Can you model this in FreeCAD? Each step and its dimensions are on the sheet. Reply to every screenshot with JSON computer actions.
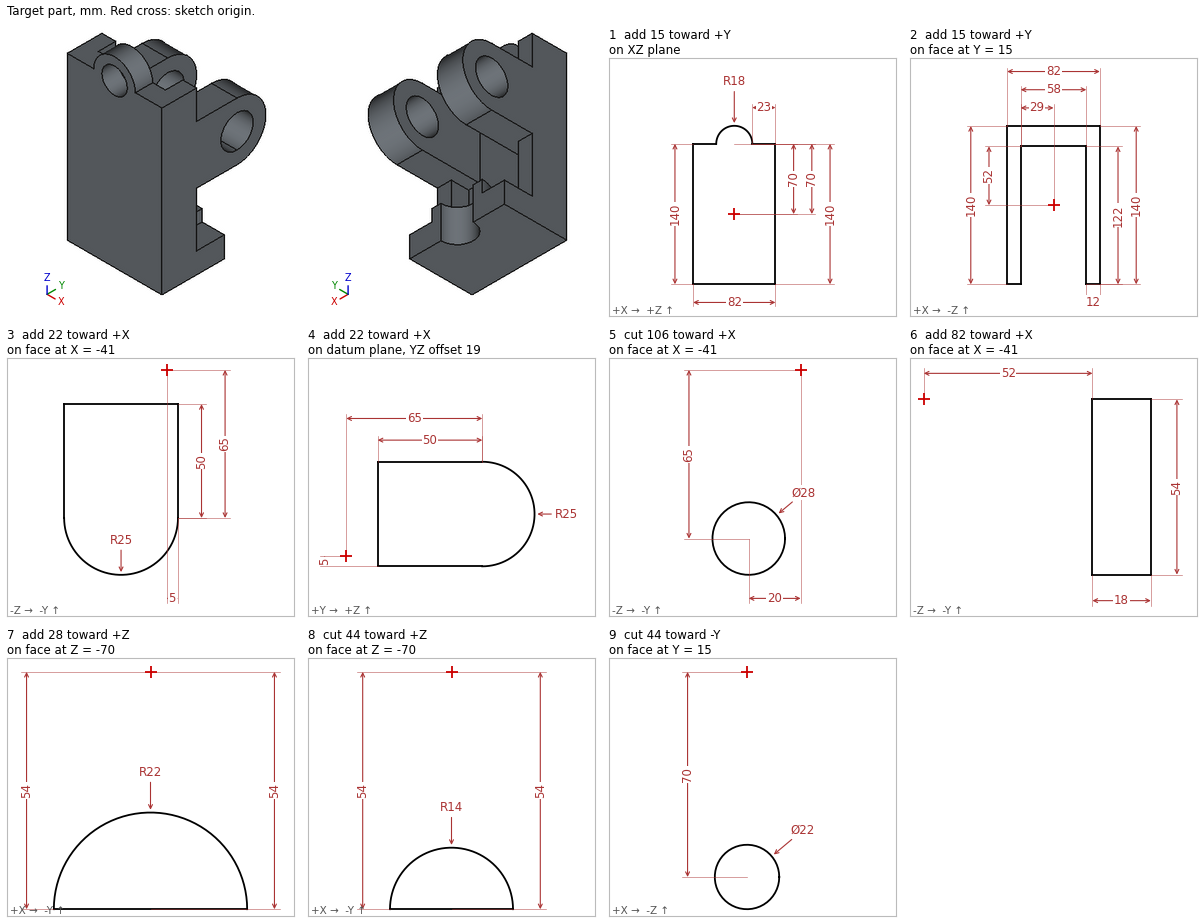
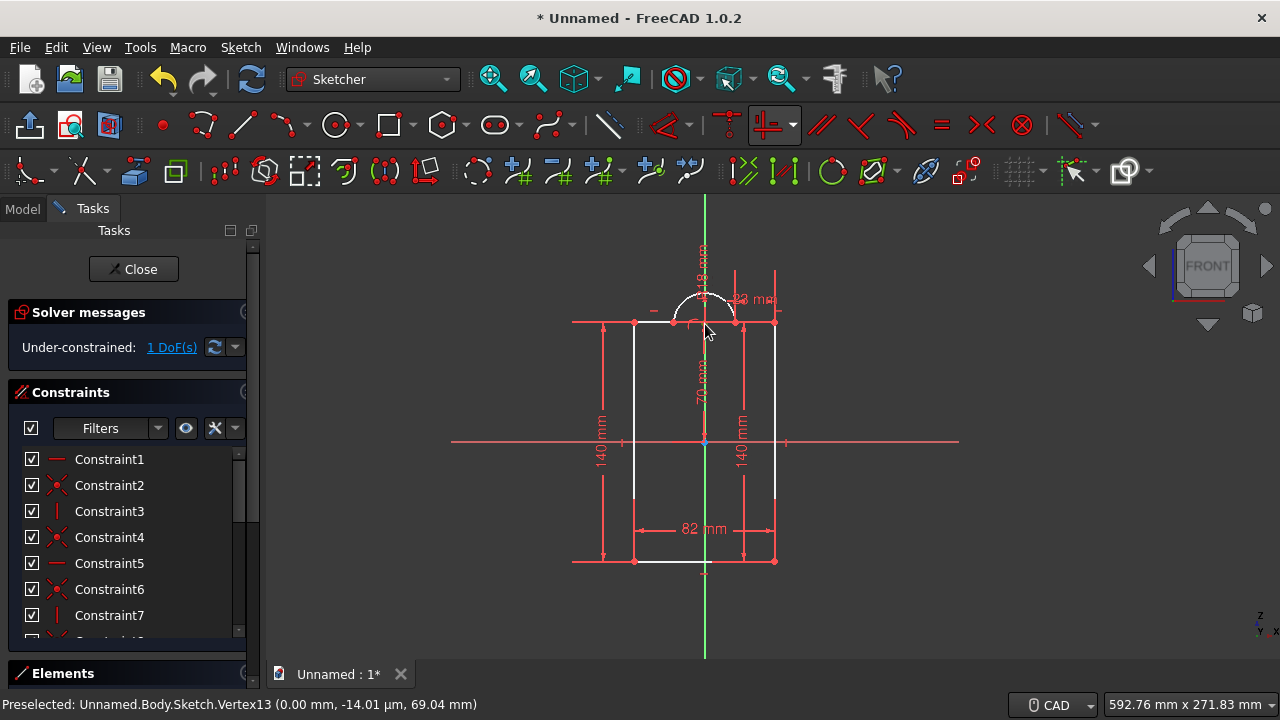
{"action": "left_click", "coordinate": [692, 126]}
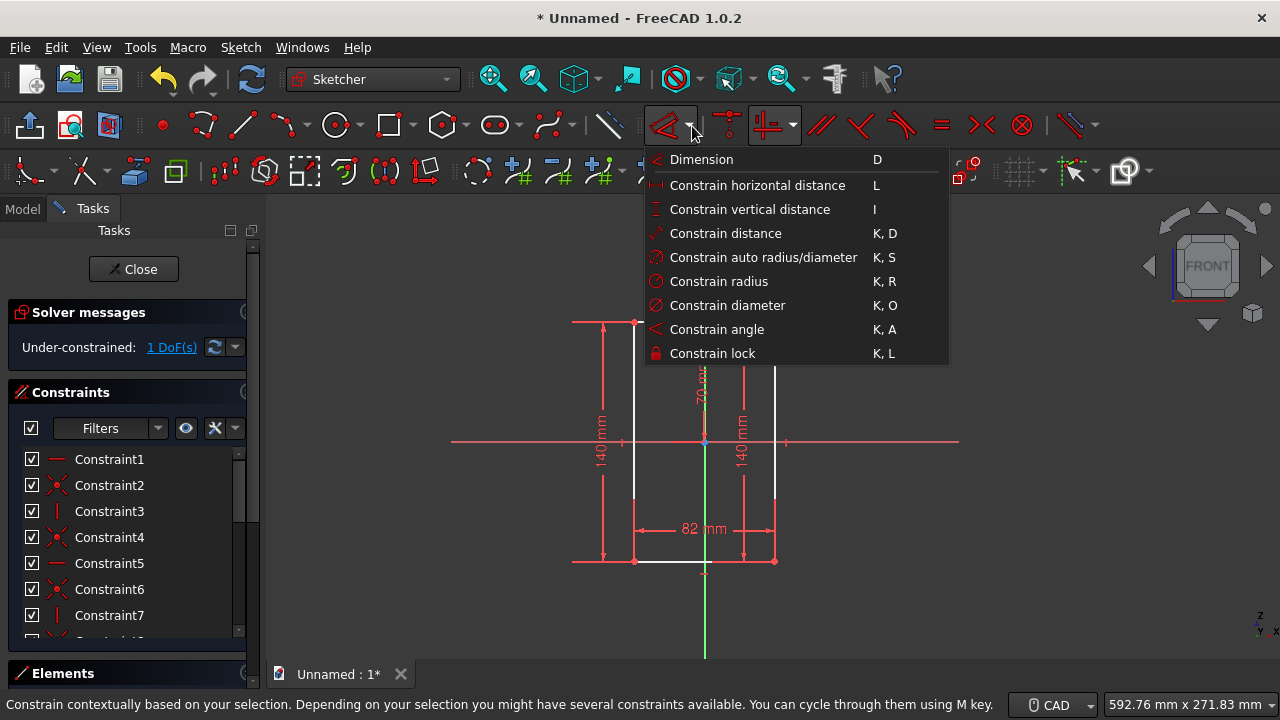
{"action": "left_click", "coordinate": [797, 209]}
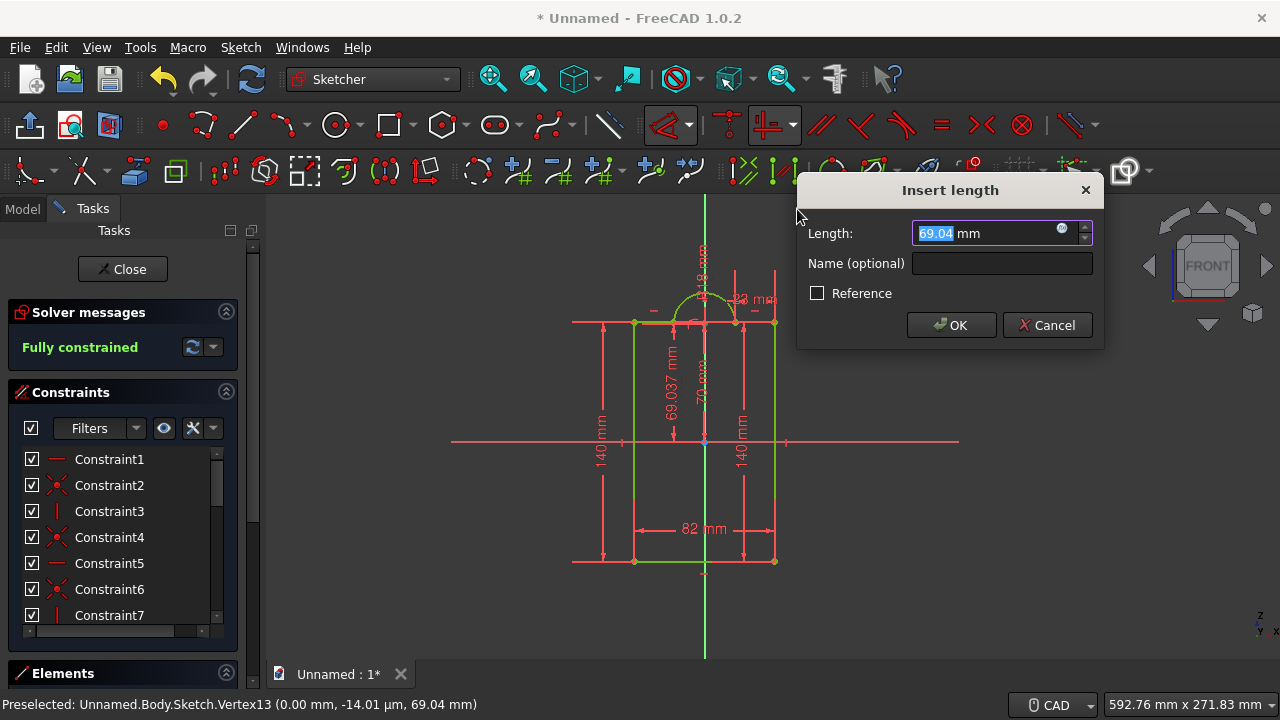
{"action": "type", "text": "70"}
{"action": "key", "text": "Return"}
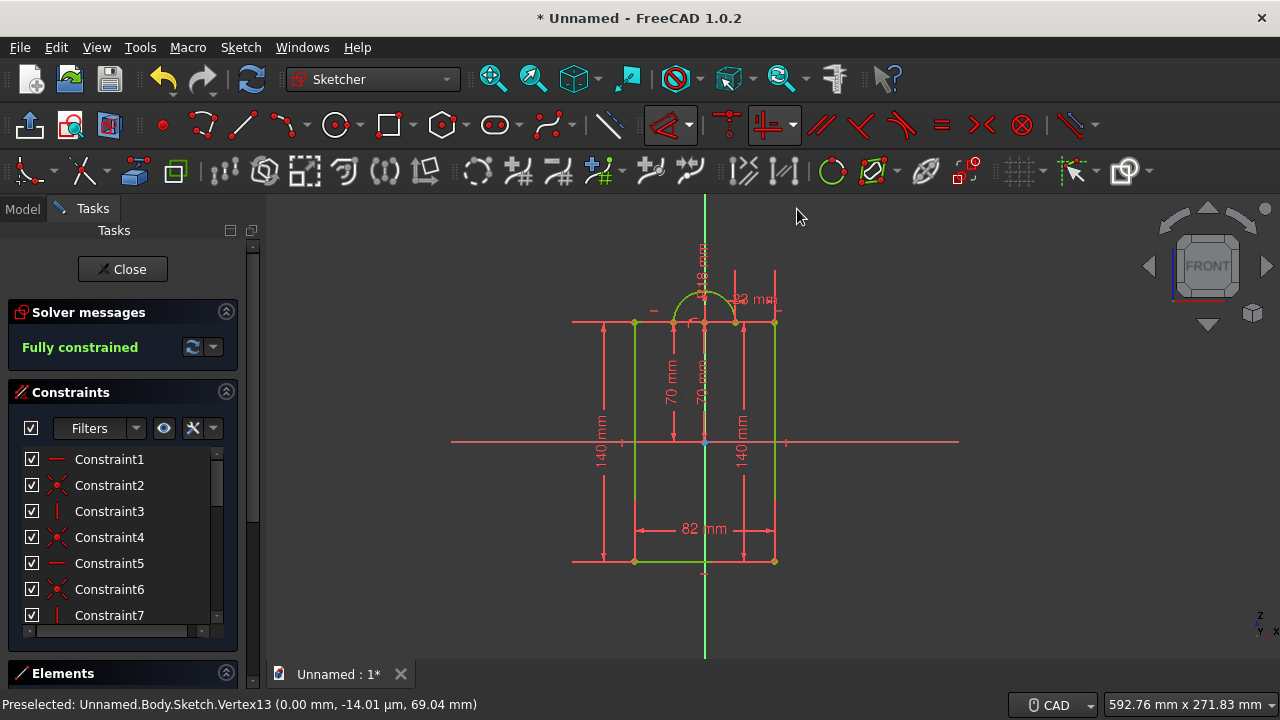
{"action": "left_click", "coordinate": [123, 269]}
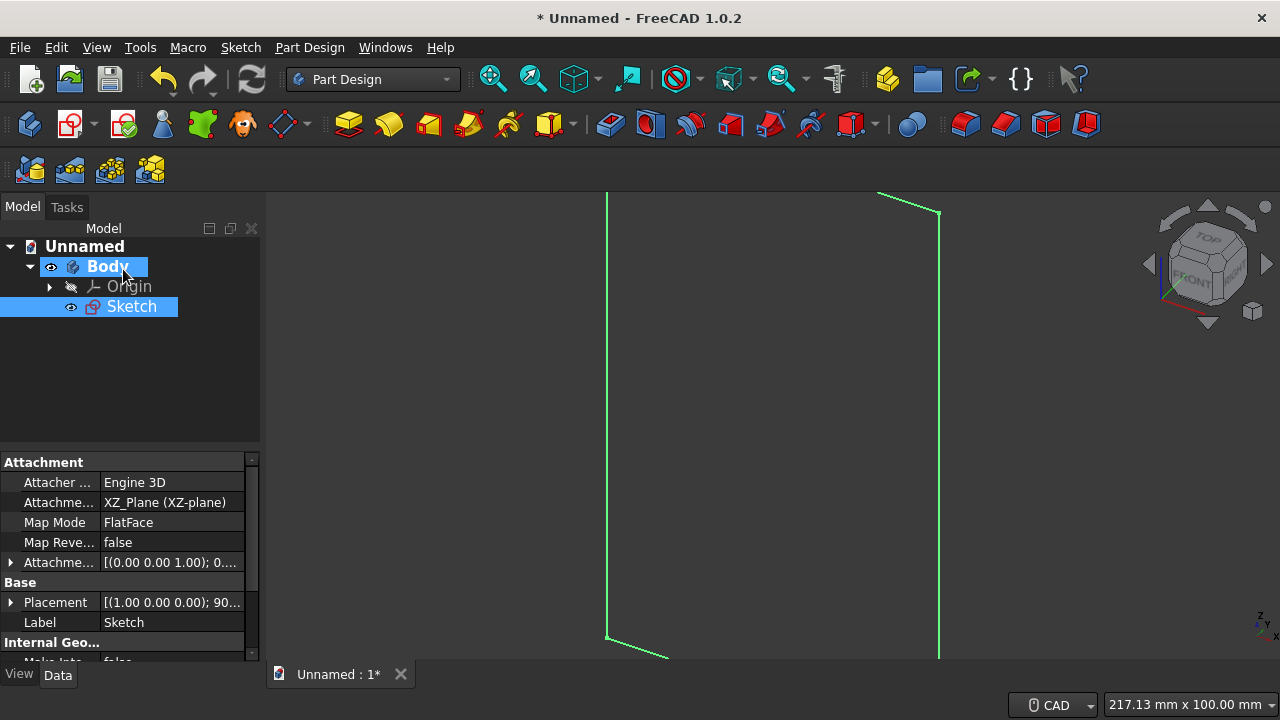
{"action": "left_click", "coordinate": [350, 124]}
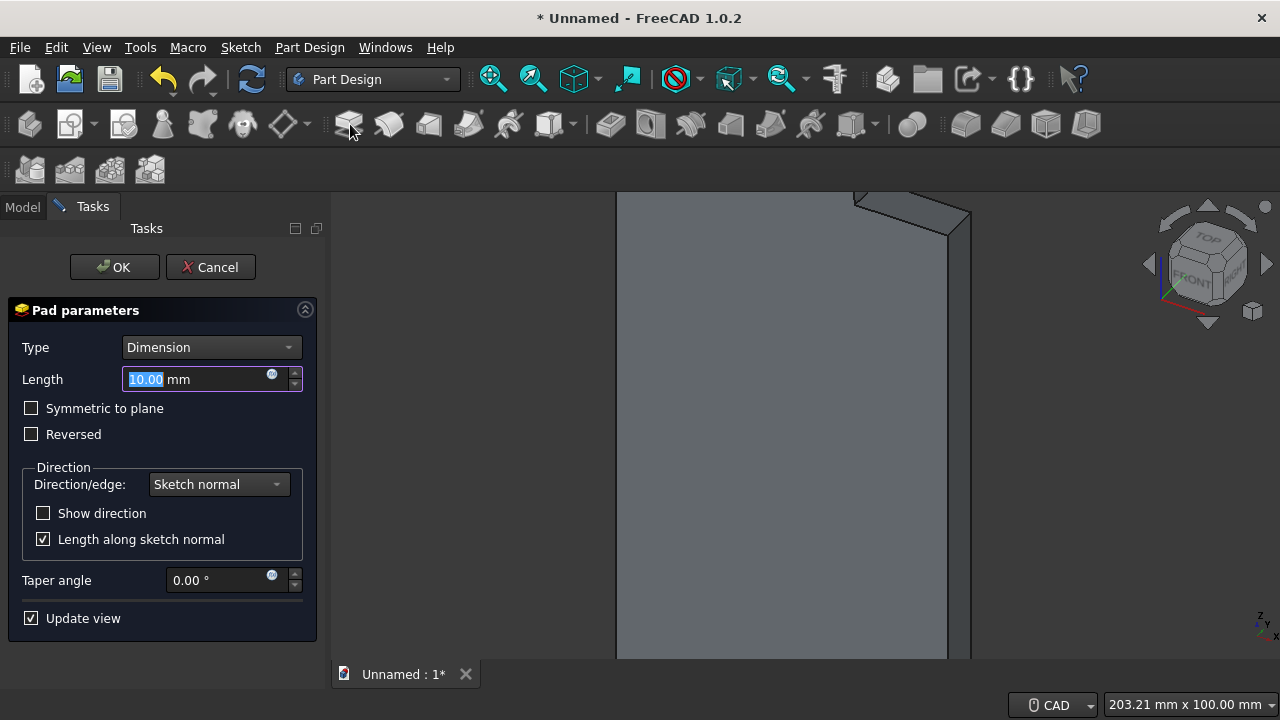
{"action": "type", "text": "15"}
{"action": "key", "text": "Tab"}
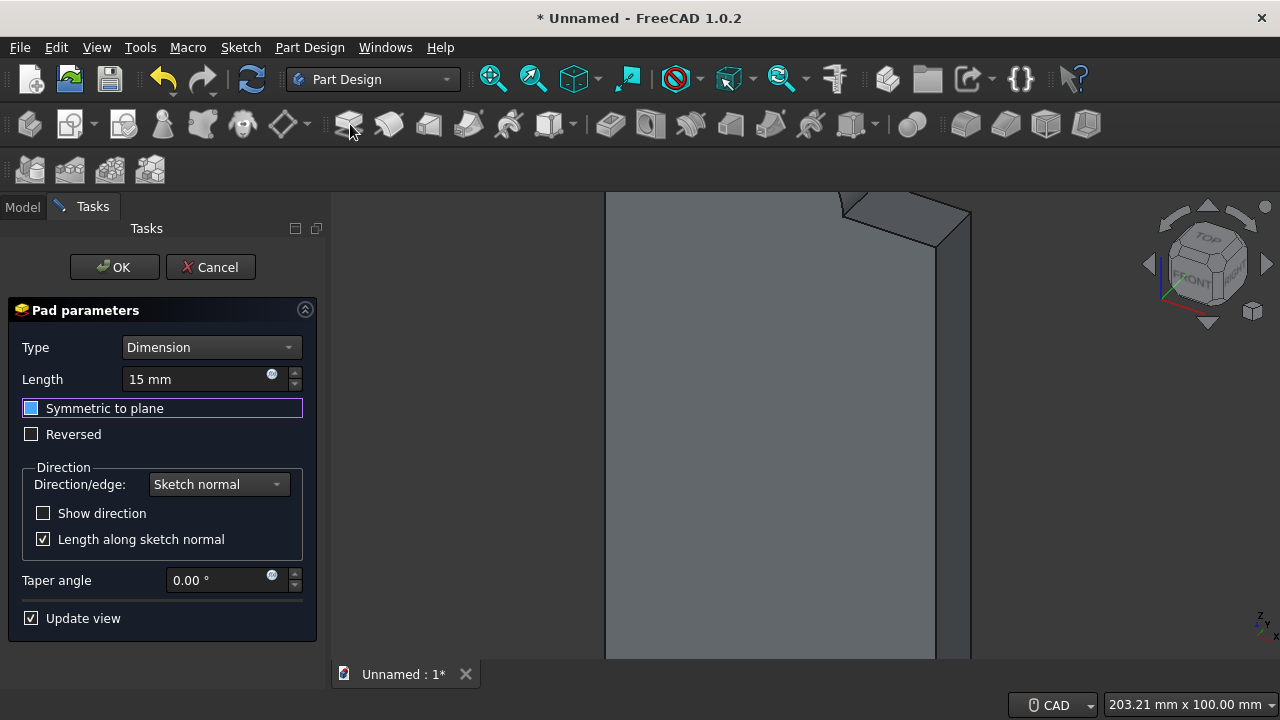
{"action": "left_click", "coordinate": [30, 434]}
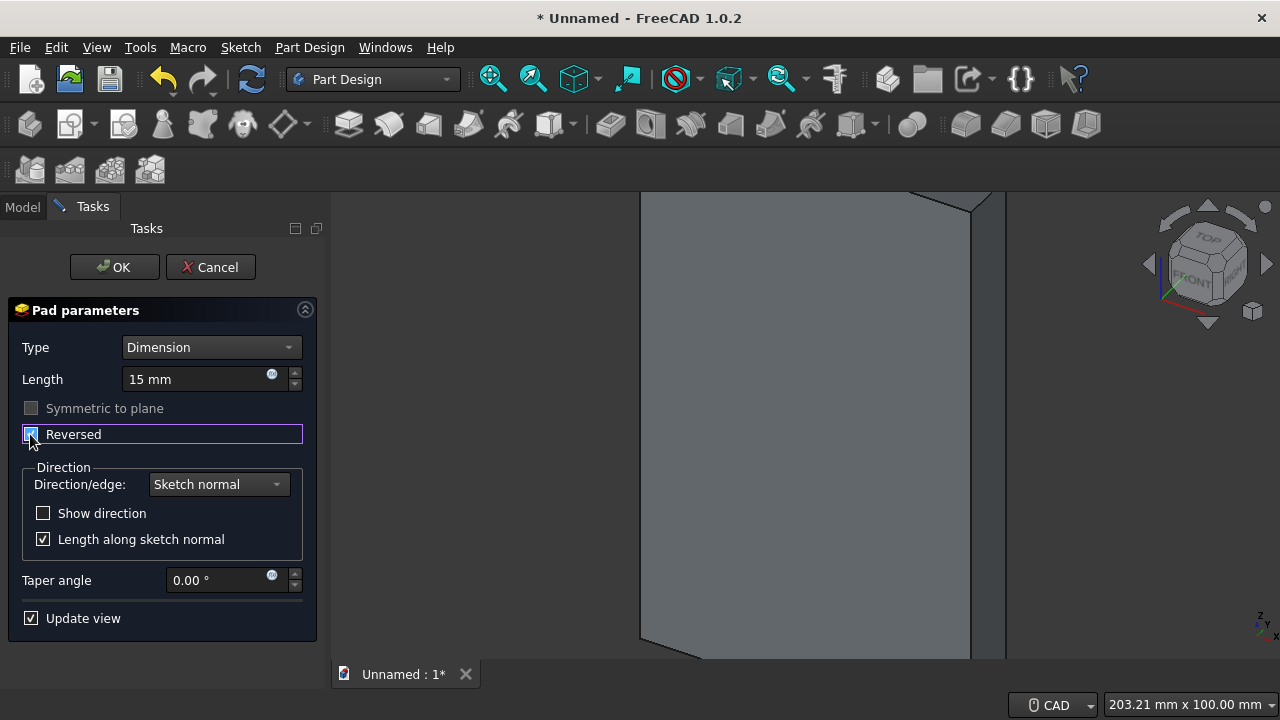
{"action": "left_click", "coordinate": [115, 267]}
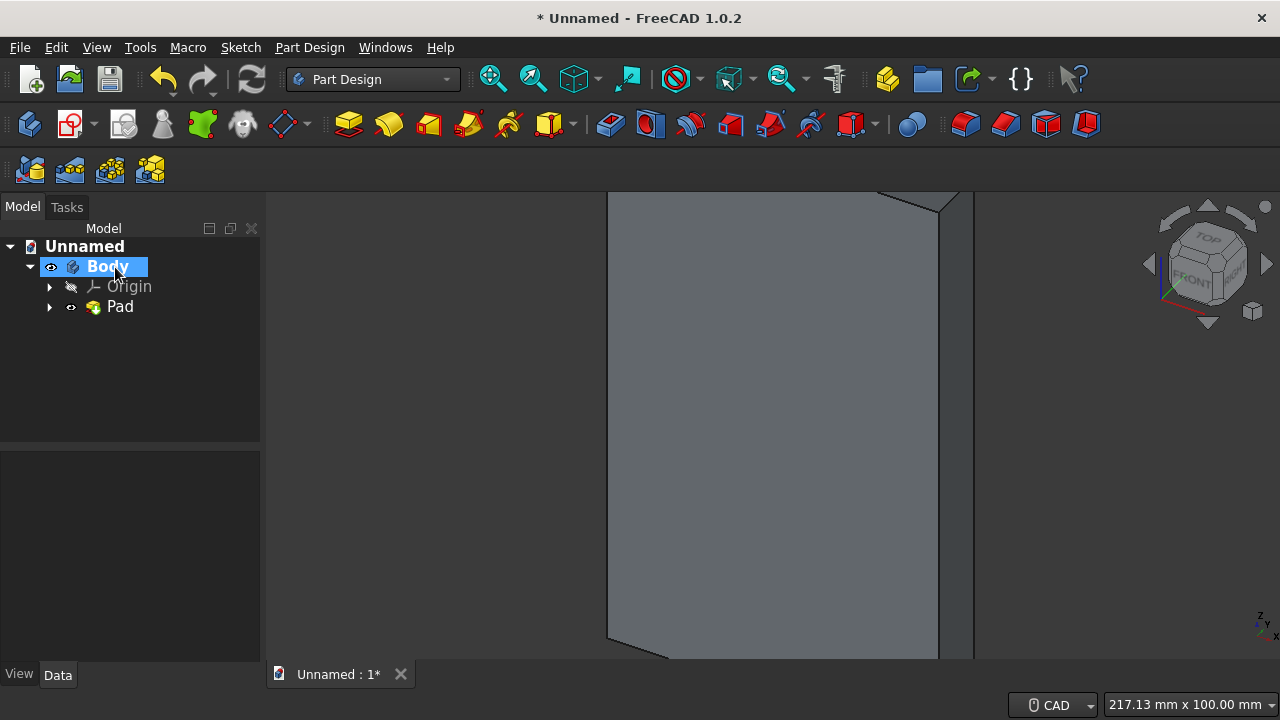
{"action": "left_click", "coordinate": [494, 80]}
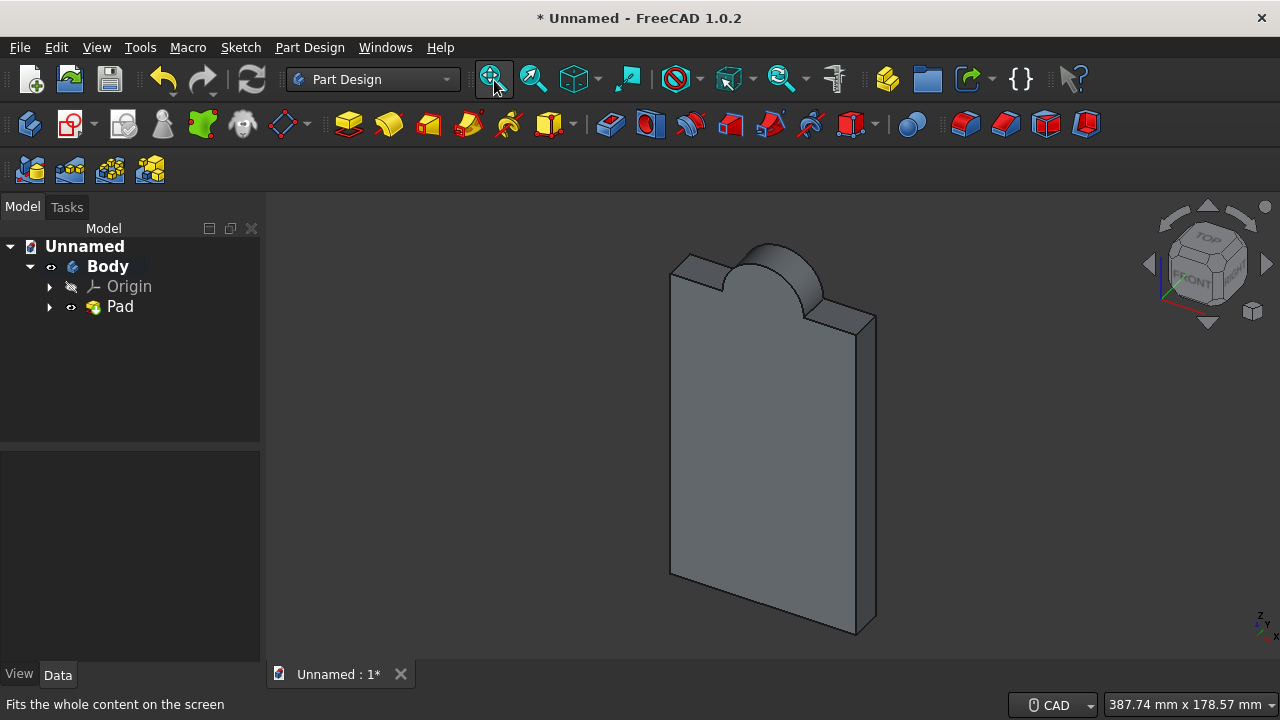
{"action": "key", "text": "4"}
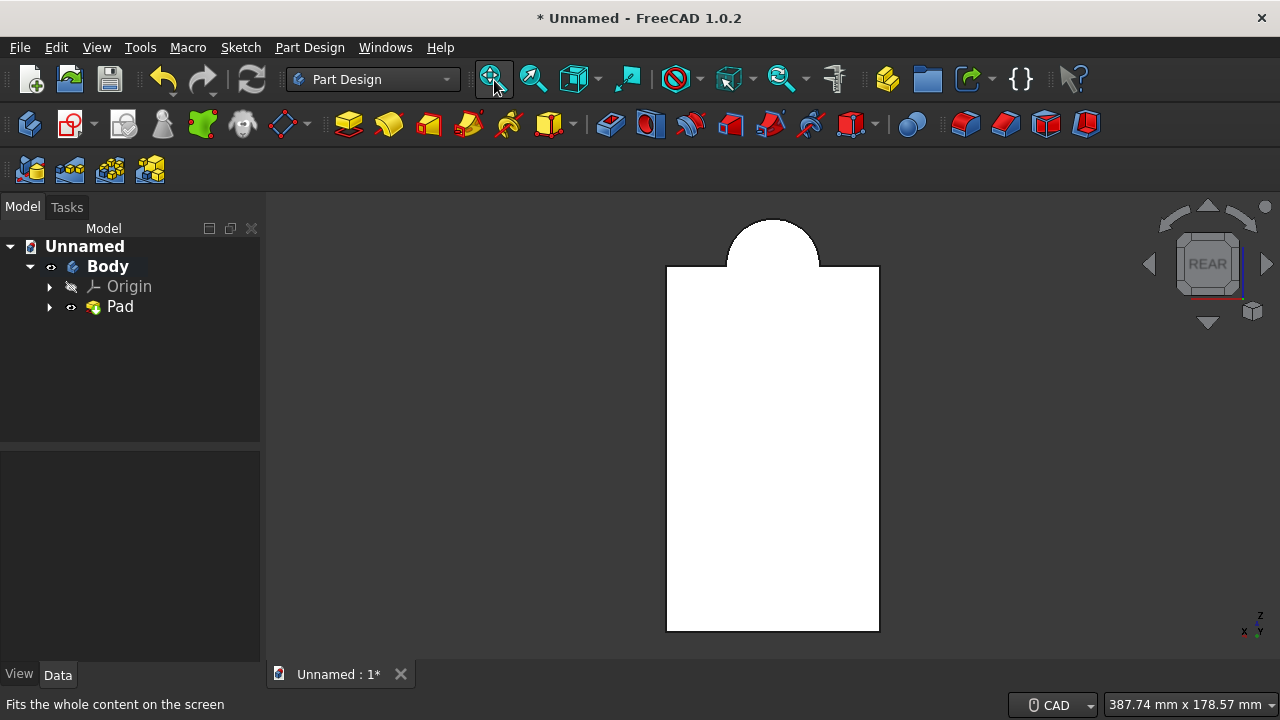
{"action": "left_click", "coordinate": [773, 365]}